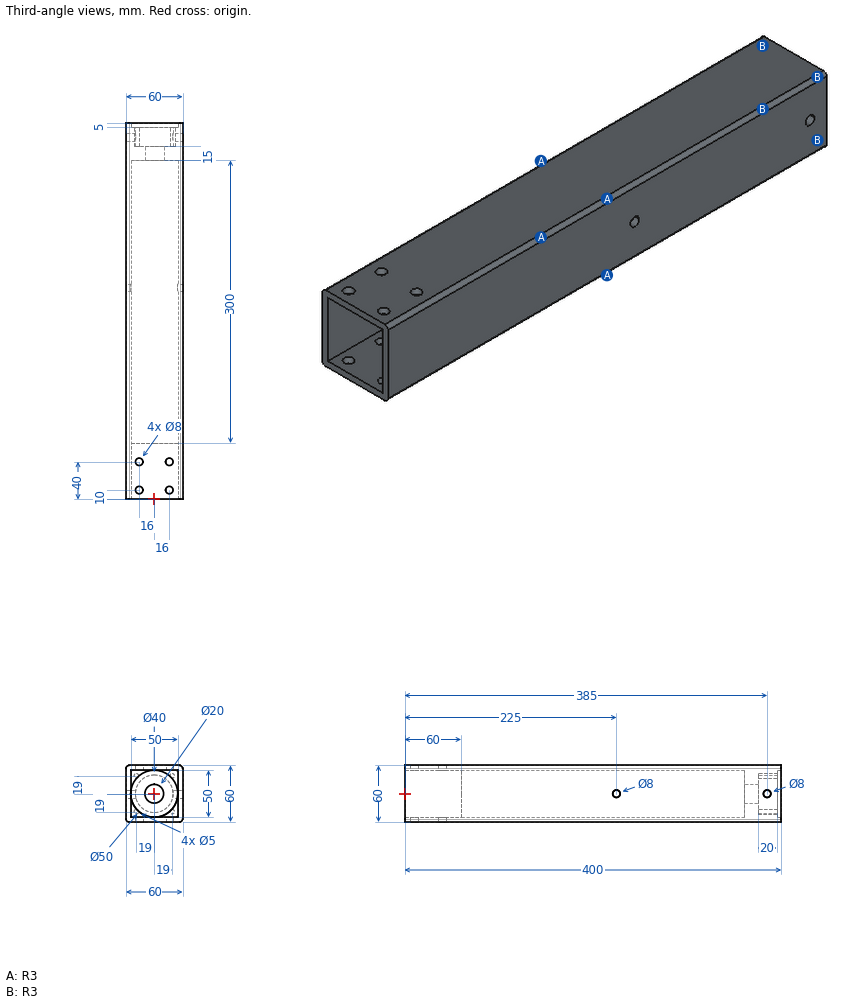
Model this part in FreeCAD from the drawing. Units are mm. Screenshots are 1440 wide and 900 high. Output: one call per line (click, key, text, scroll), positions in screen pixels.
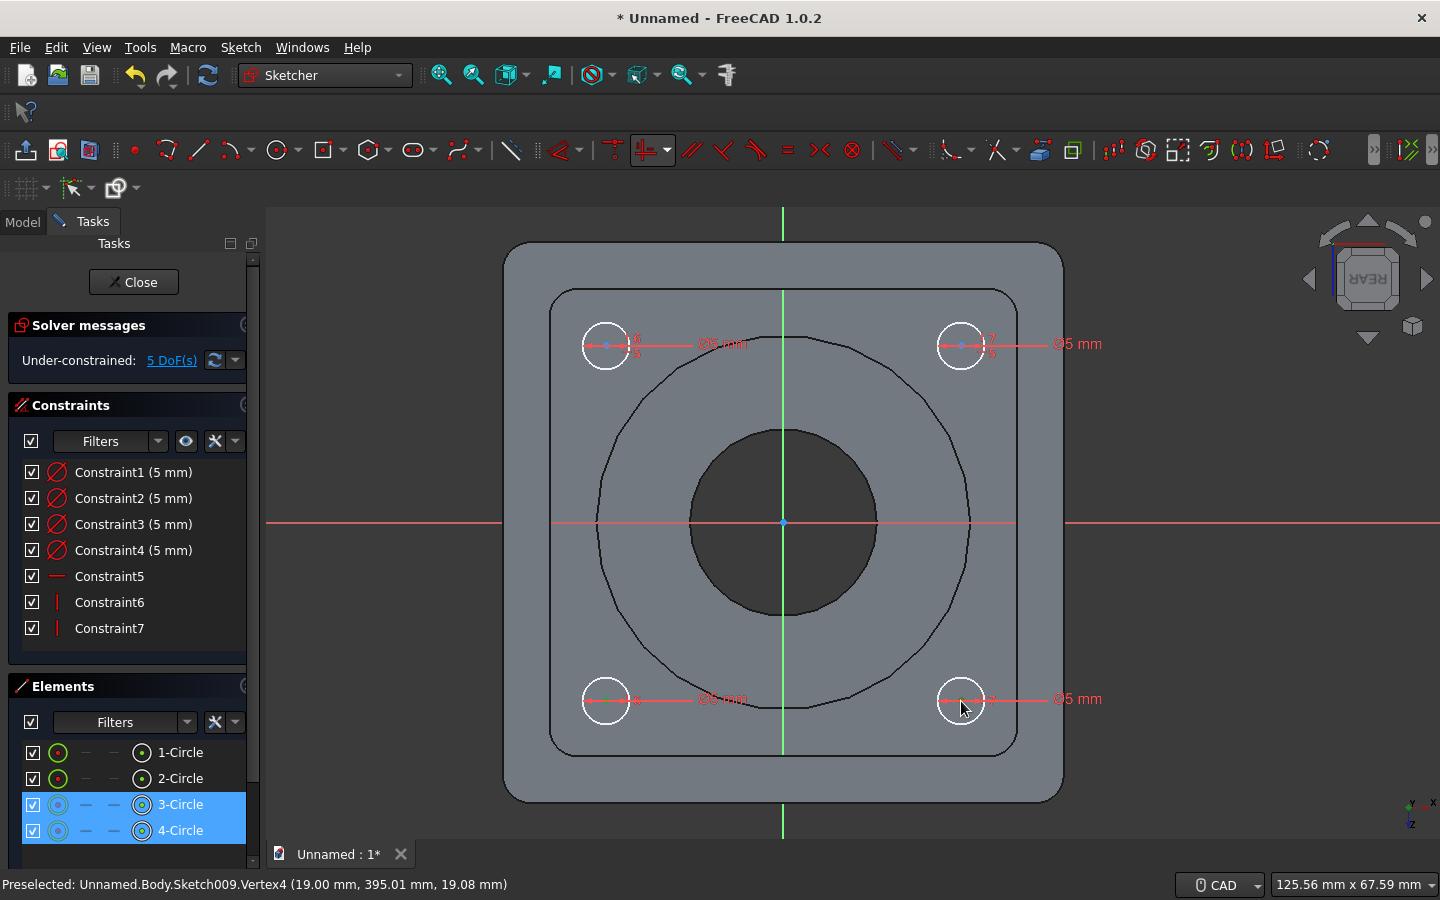
click(670, 150)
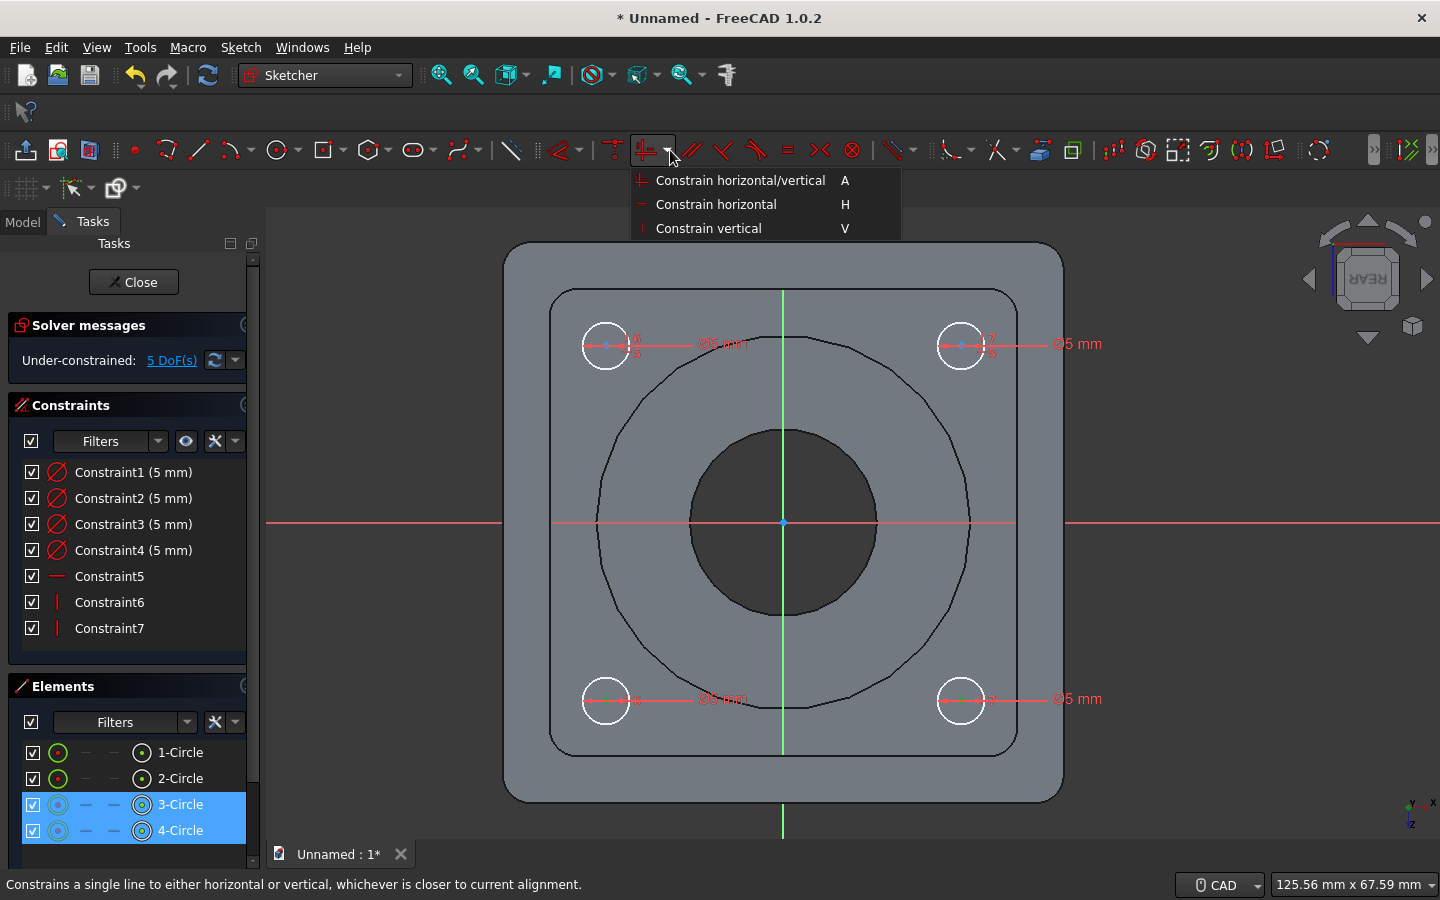
click(766, 204)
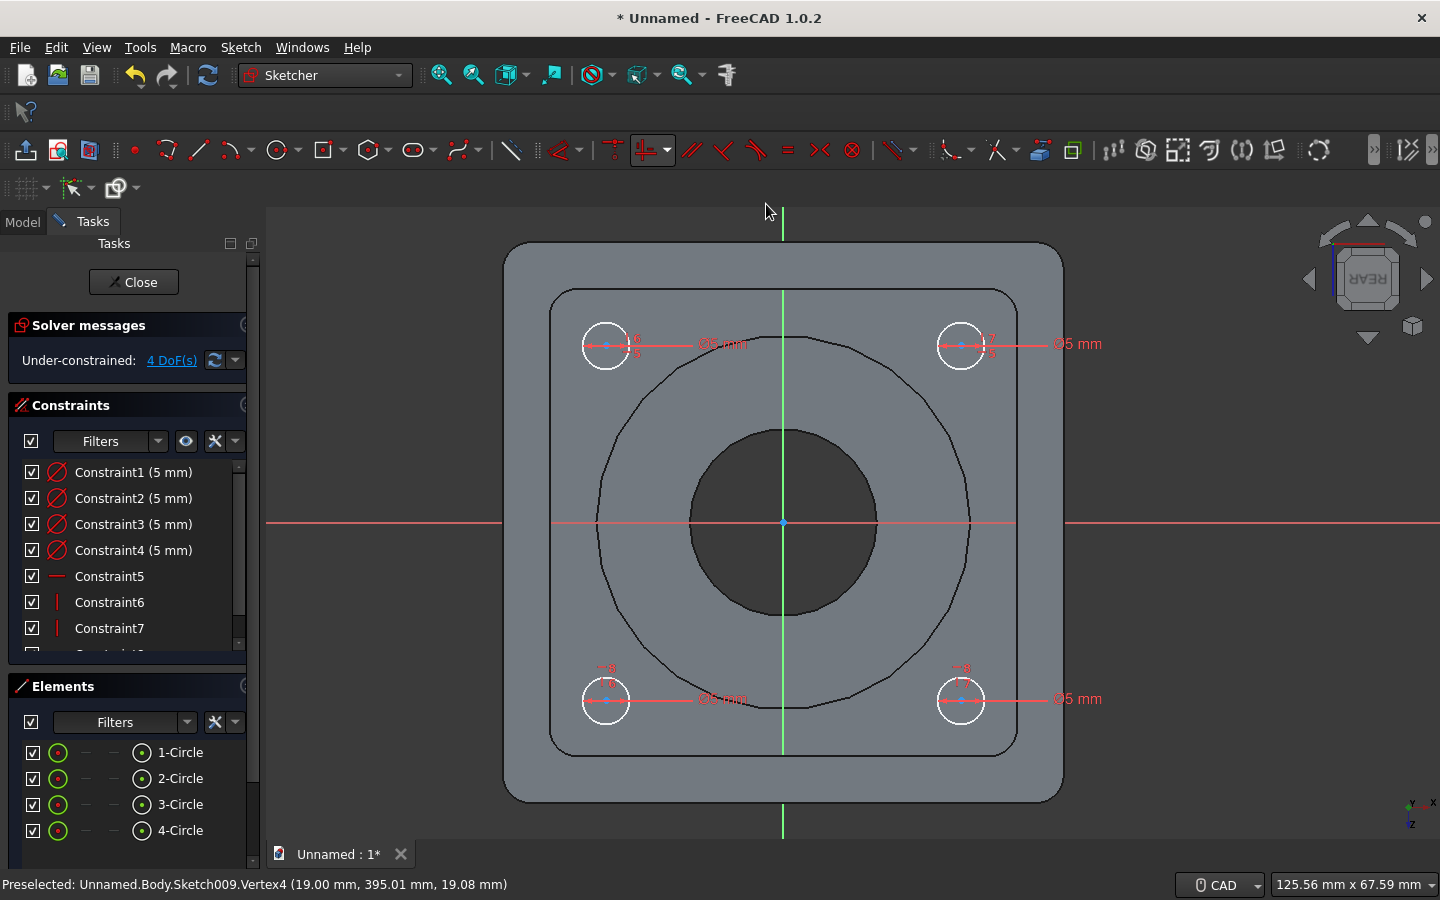
click(558, 150)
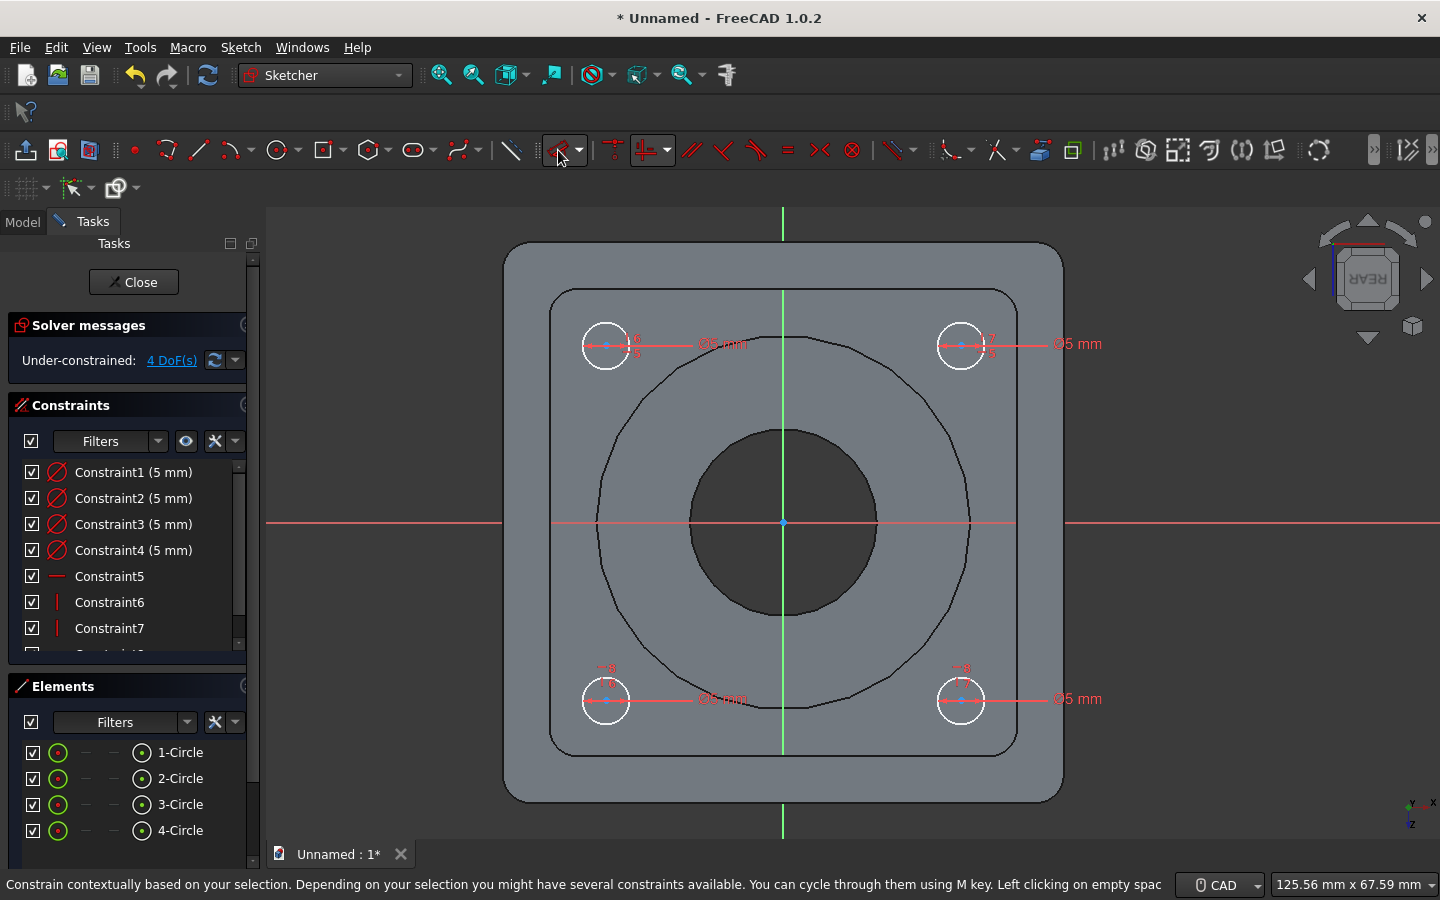
click(606, 346)
click(695, 312)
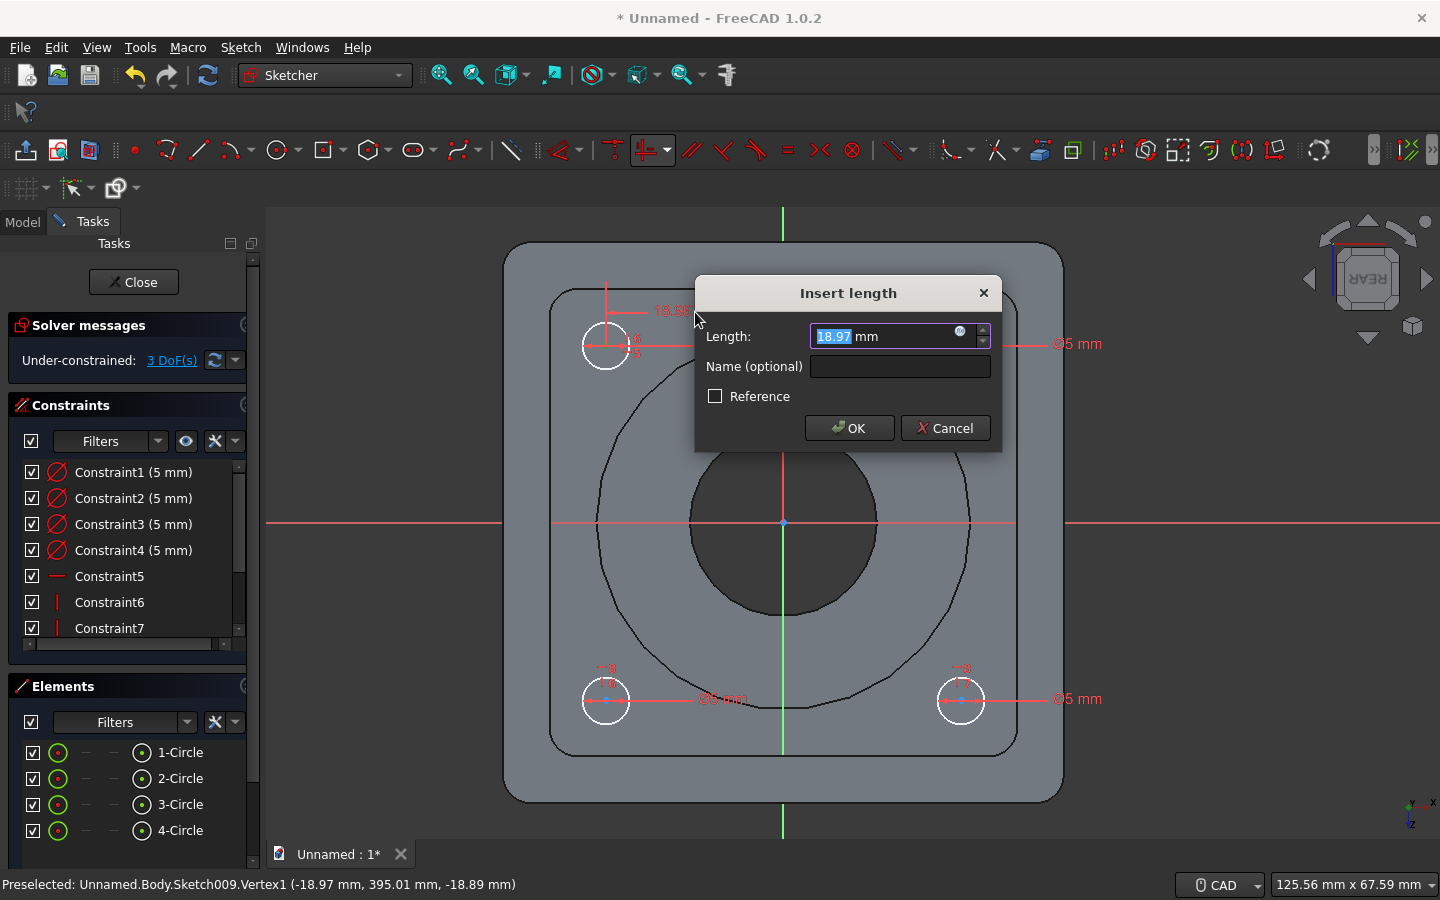
text(19)
key(Return)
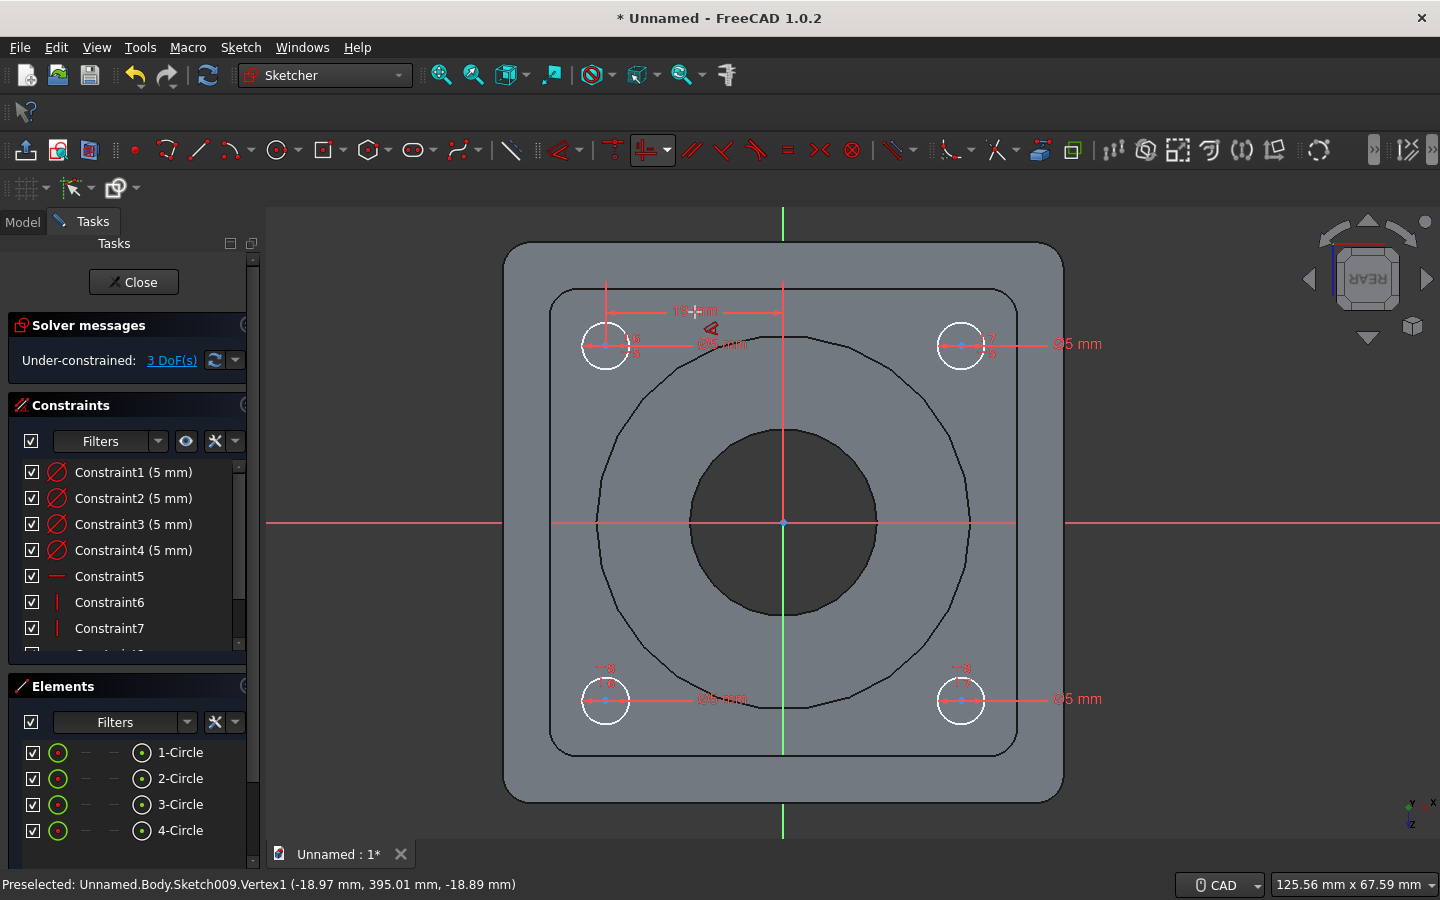
click(606, 346)
click(572, 434)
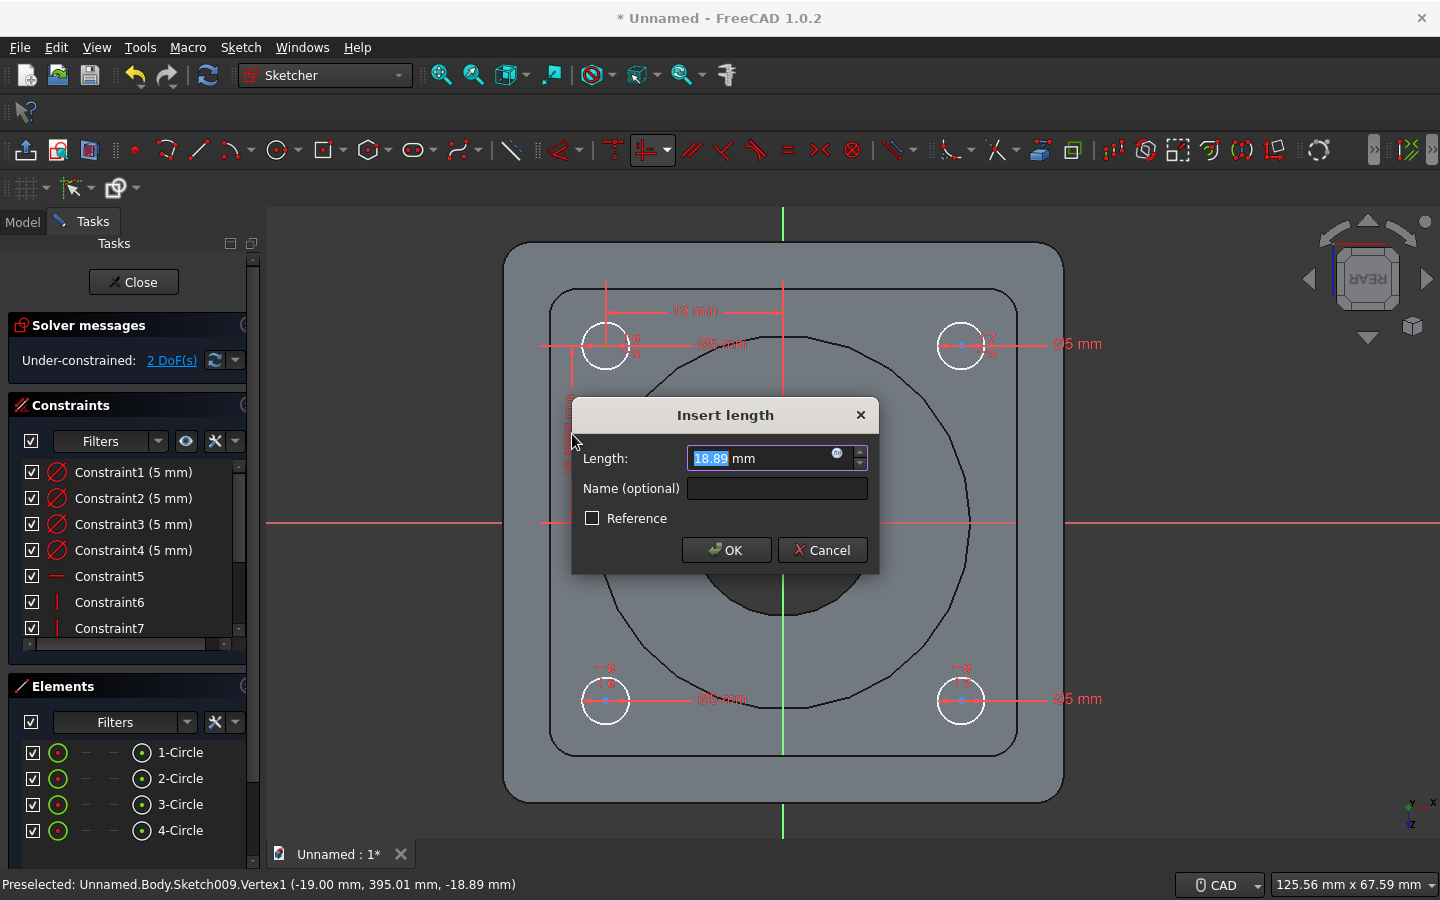
text(19)
key(Return)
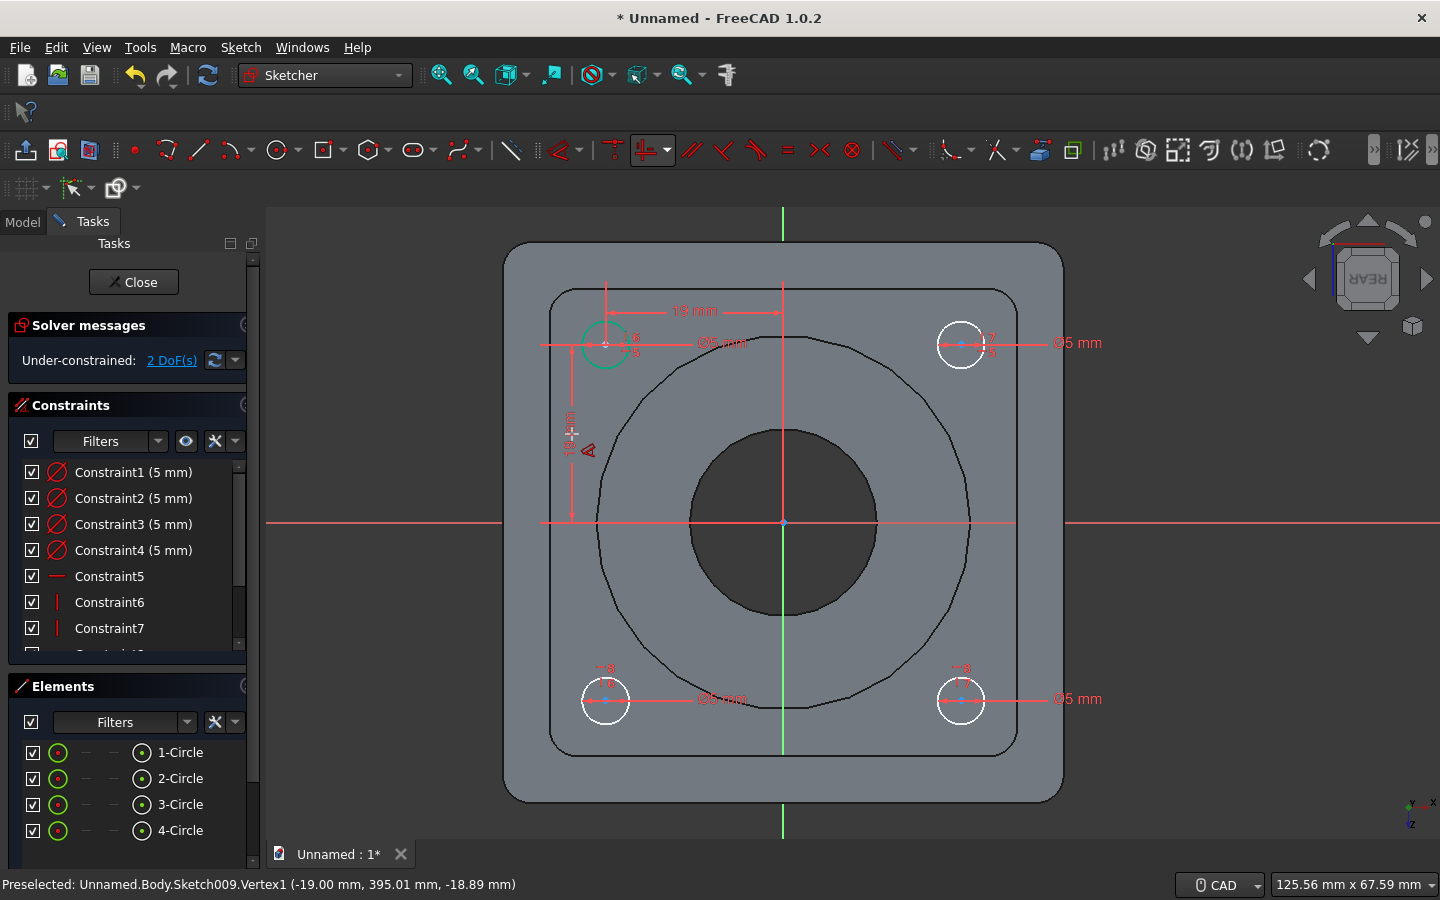
click(961, 345)
click(872, 311)